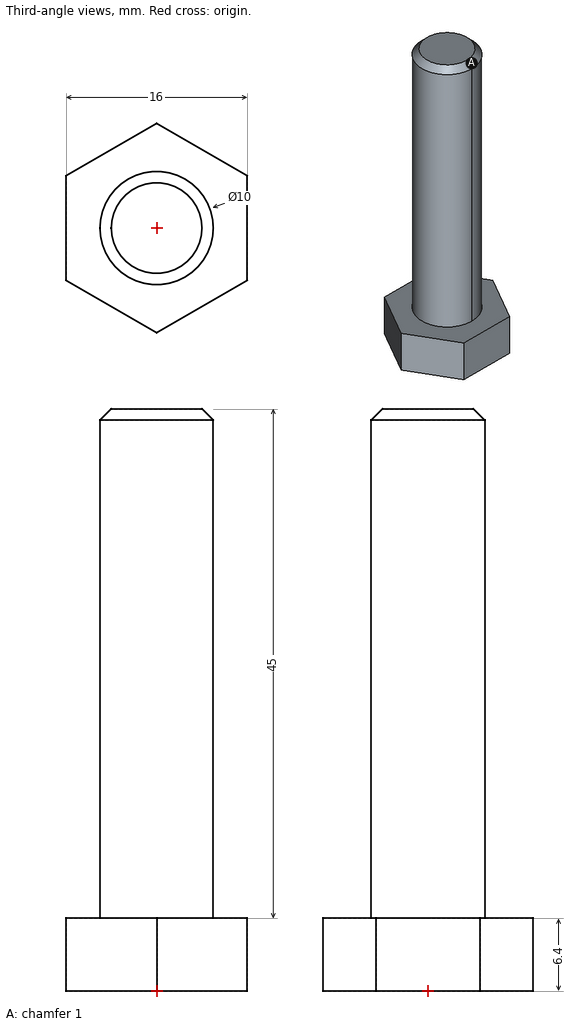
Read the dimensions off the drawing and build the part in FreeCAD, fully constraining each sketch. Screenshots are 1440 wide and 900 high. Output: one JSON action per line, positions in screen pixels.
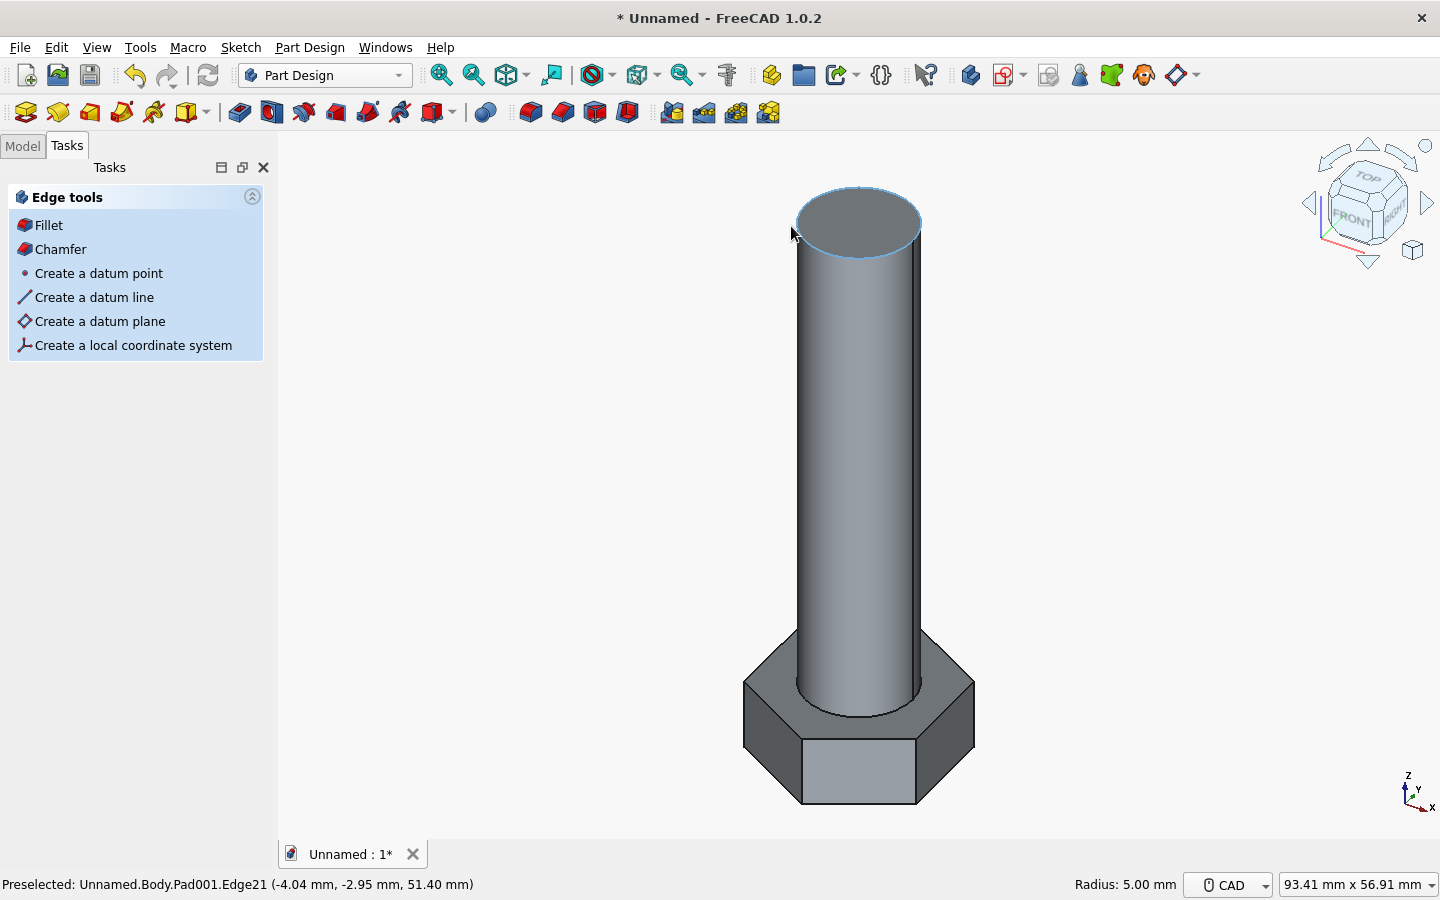
{"action": "left_click", "coordinate": [564, 112]}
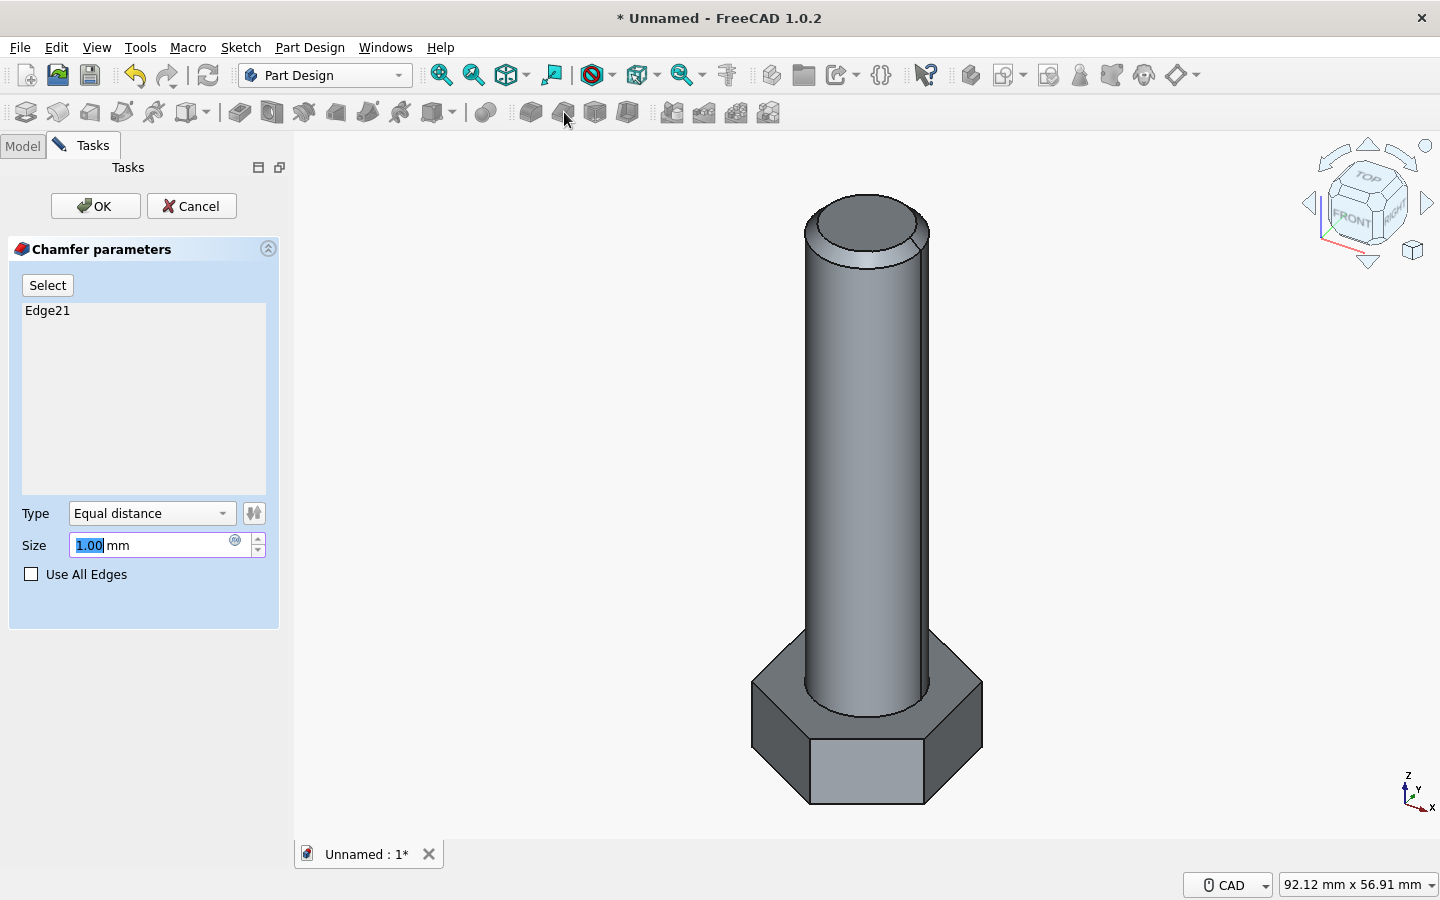
{"action": "type", "text": "1"}
{"action": "key", "text": "Tab"}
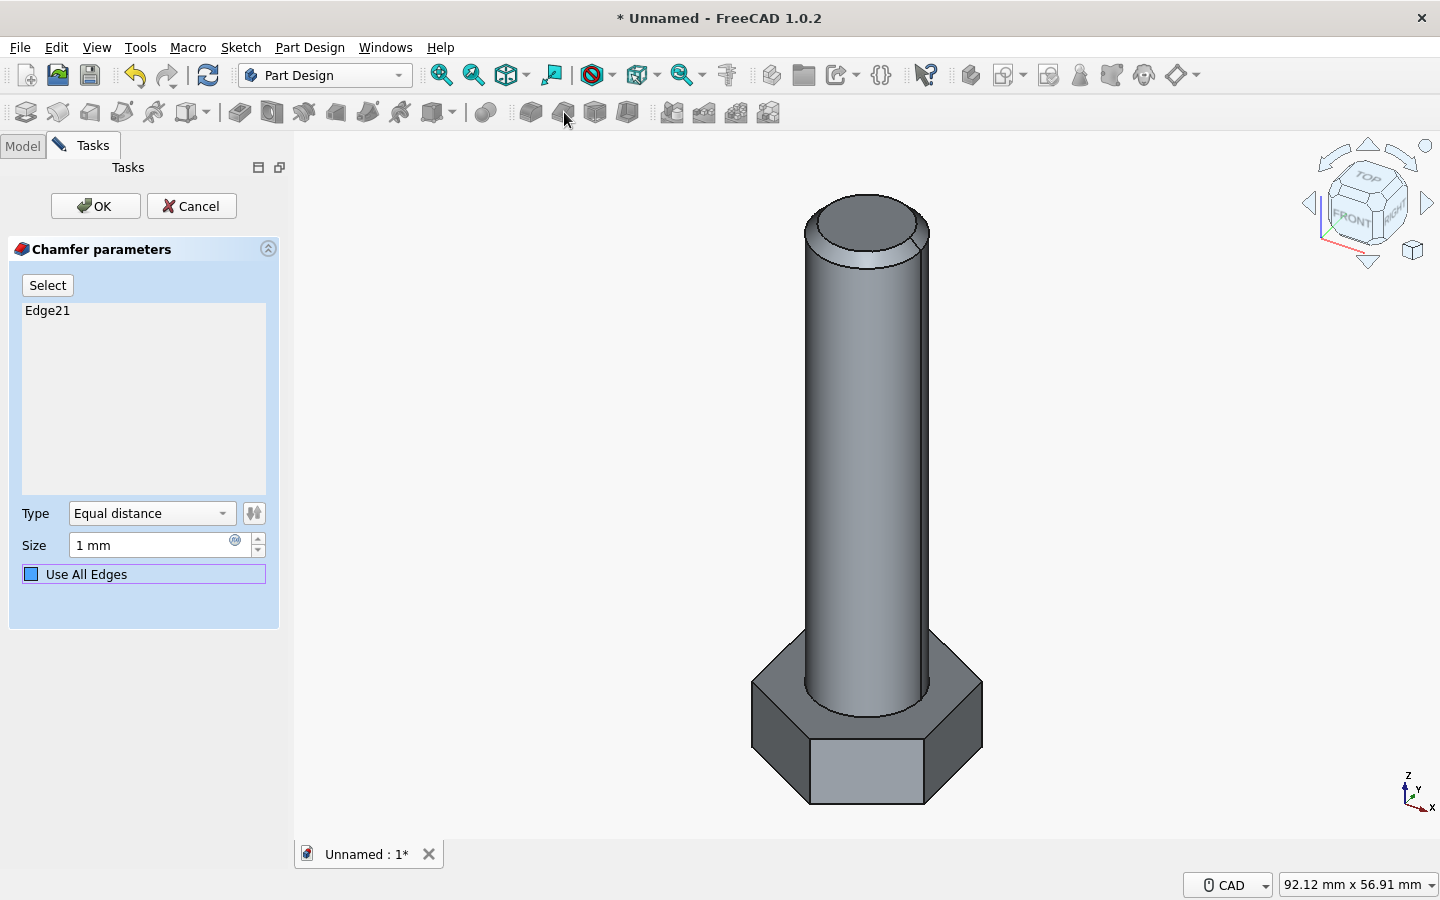
{"action": "left_click", "coordinate": [96, 206]}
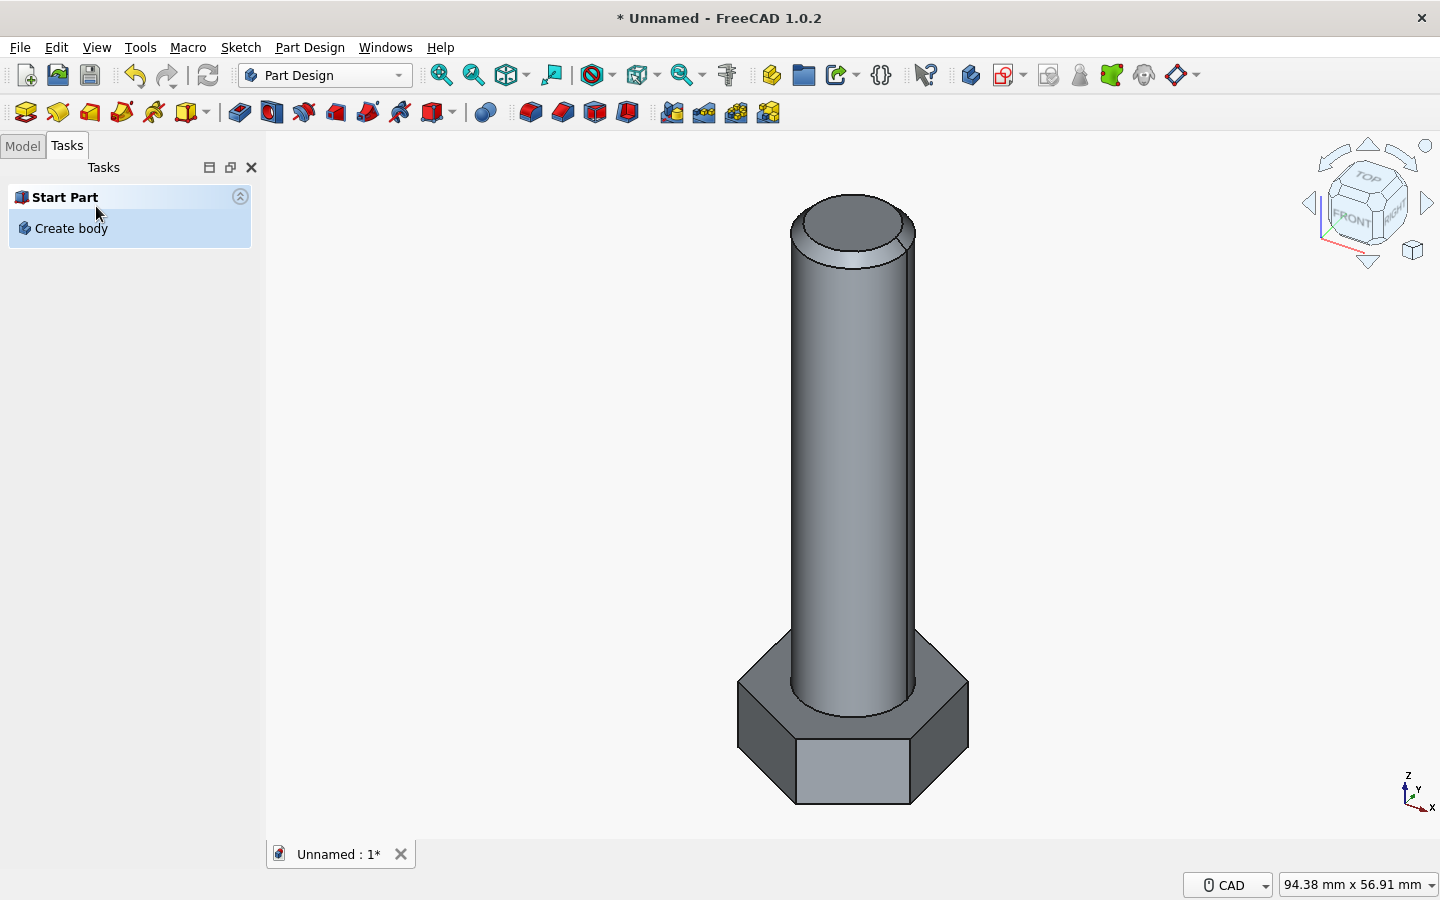
{"action": "key", "text": "0"}